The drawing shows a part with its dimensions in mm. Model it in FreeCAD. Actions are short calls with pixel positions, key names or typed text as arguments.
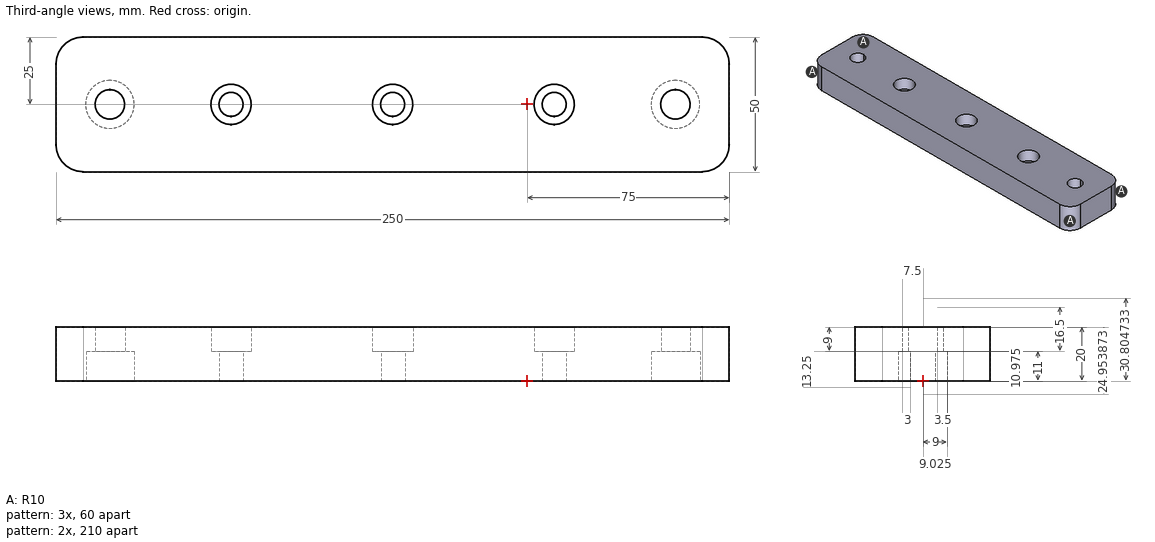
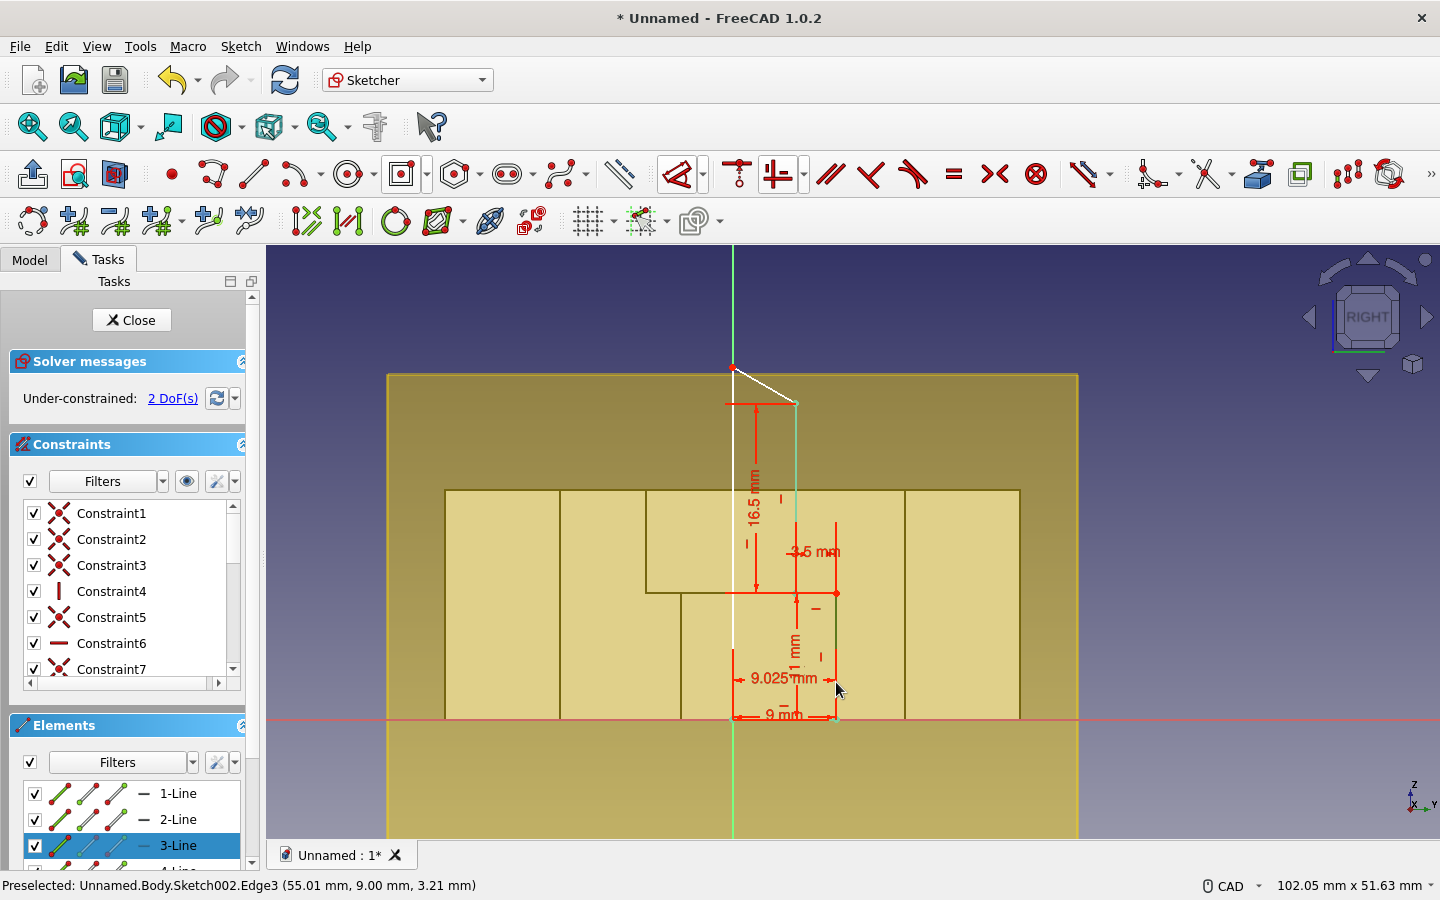
key(i)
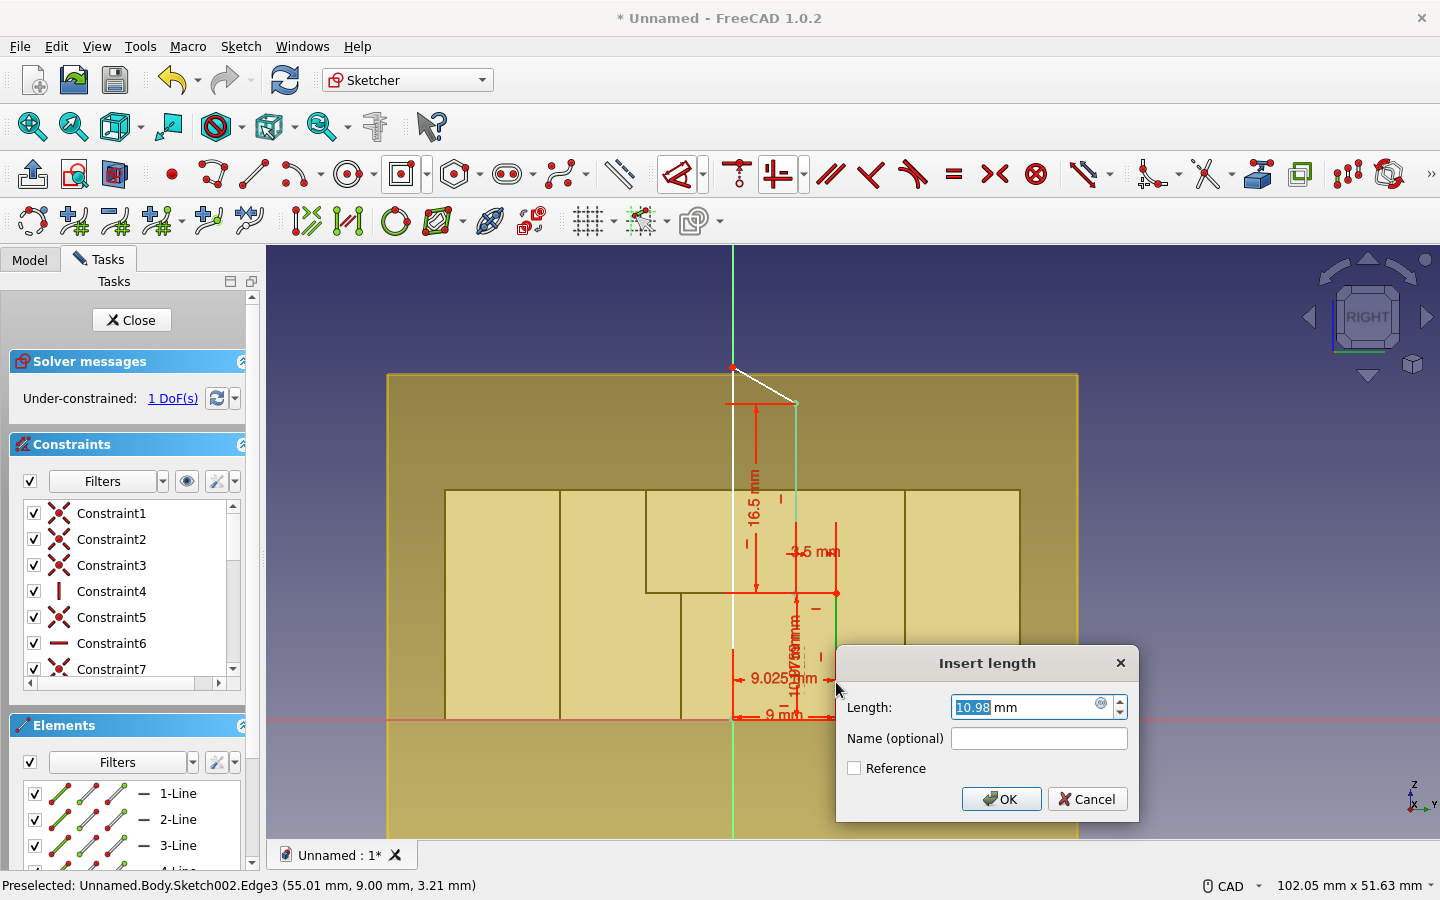
text(10.975)
key(Return)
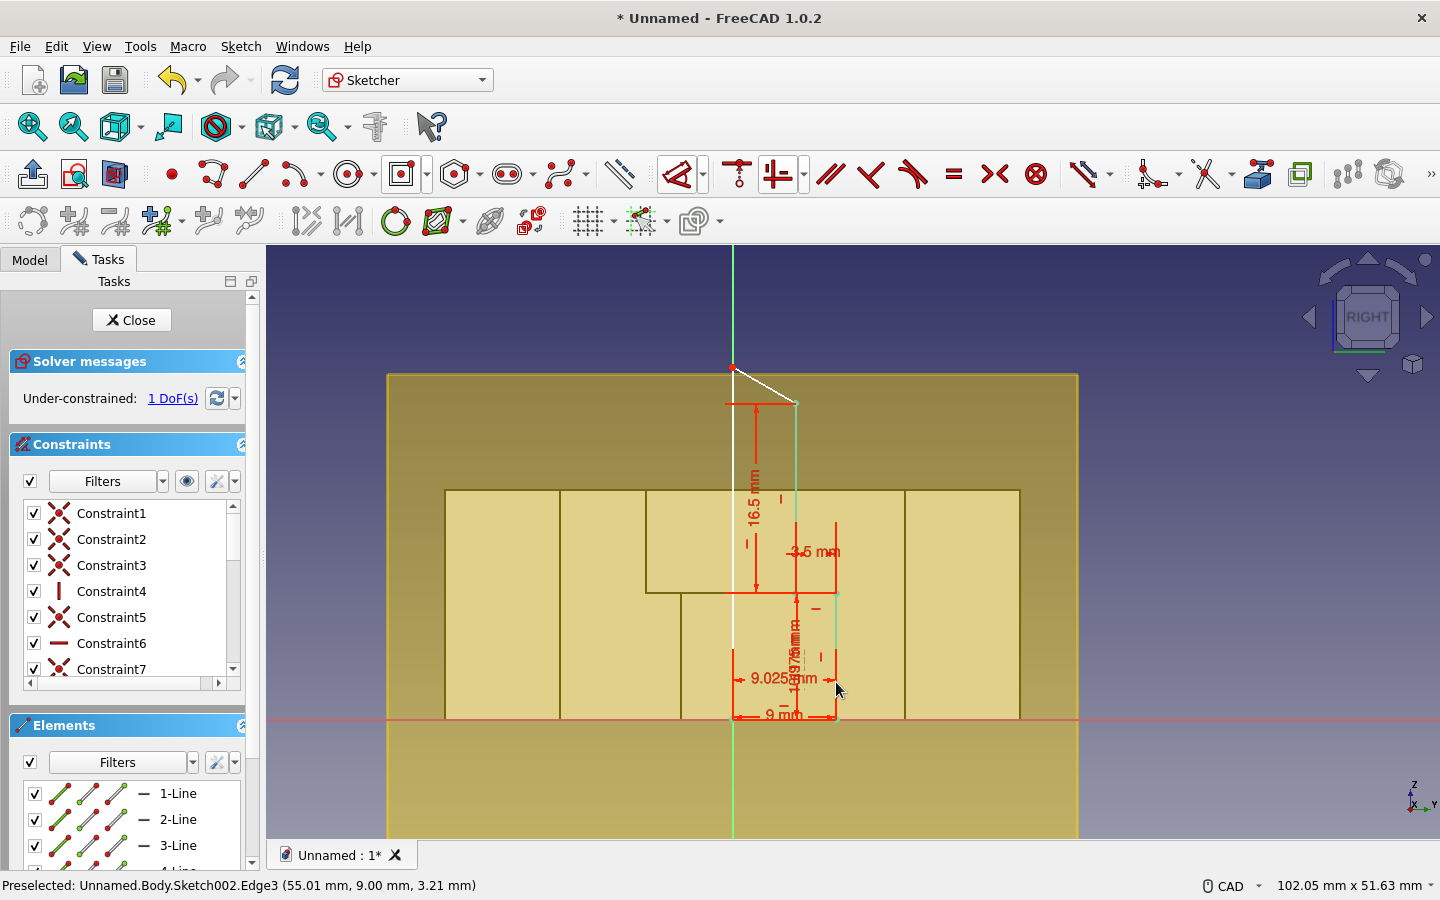
click(733, 473)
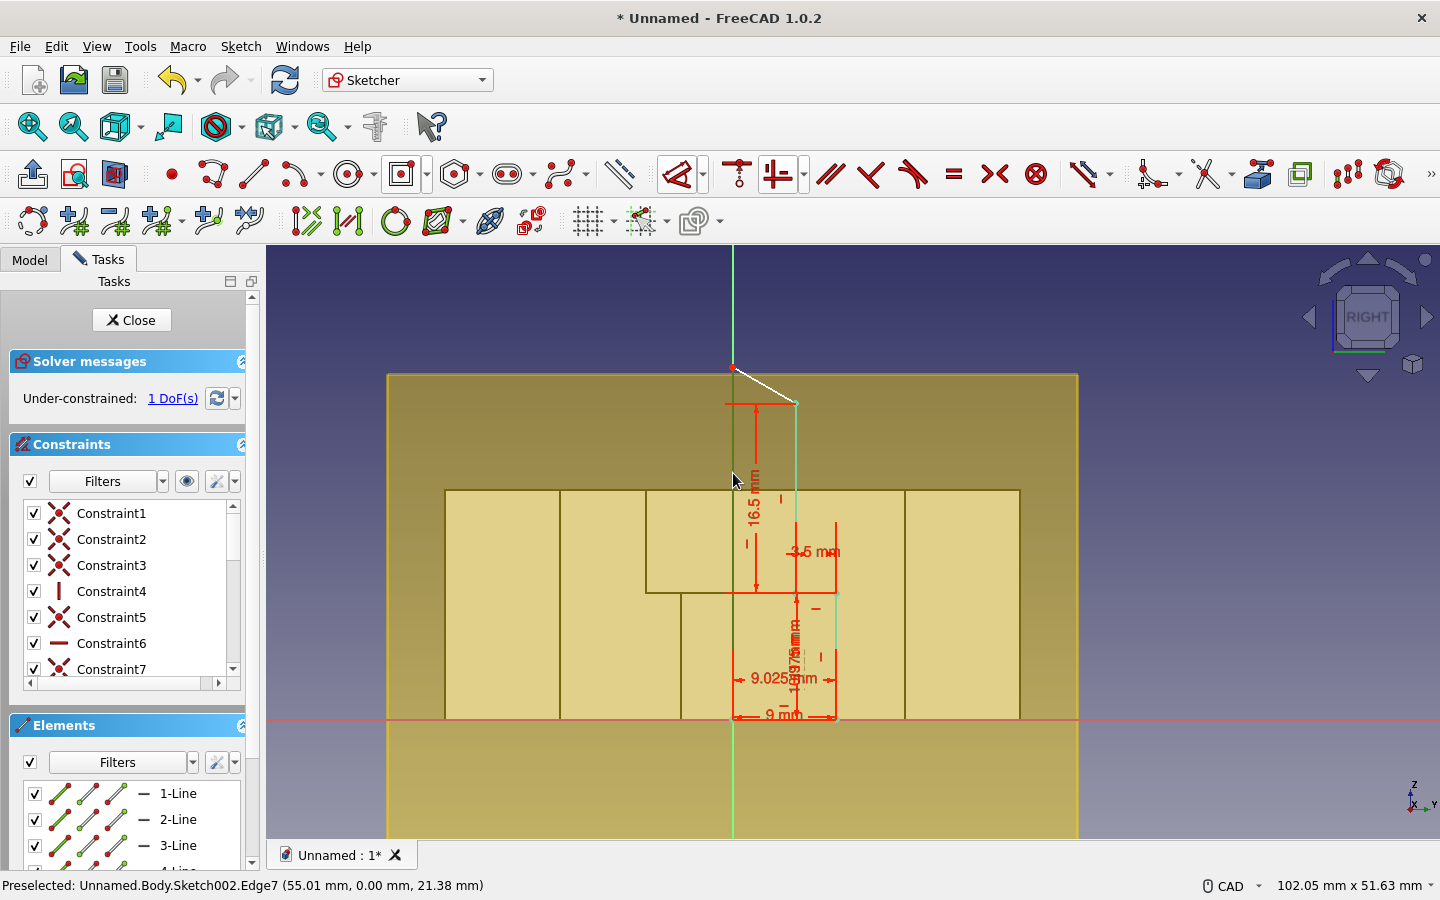
key(i)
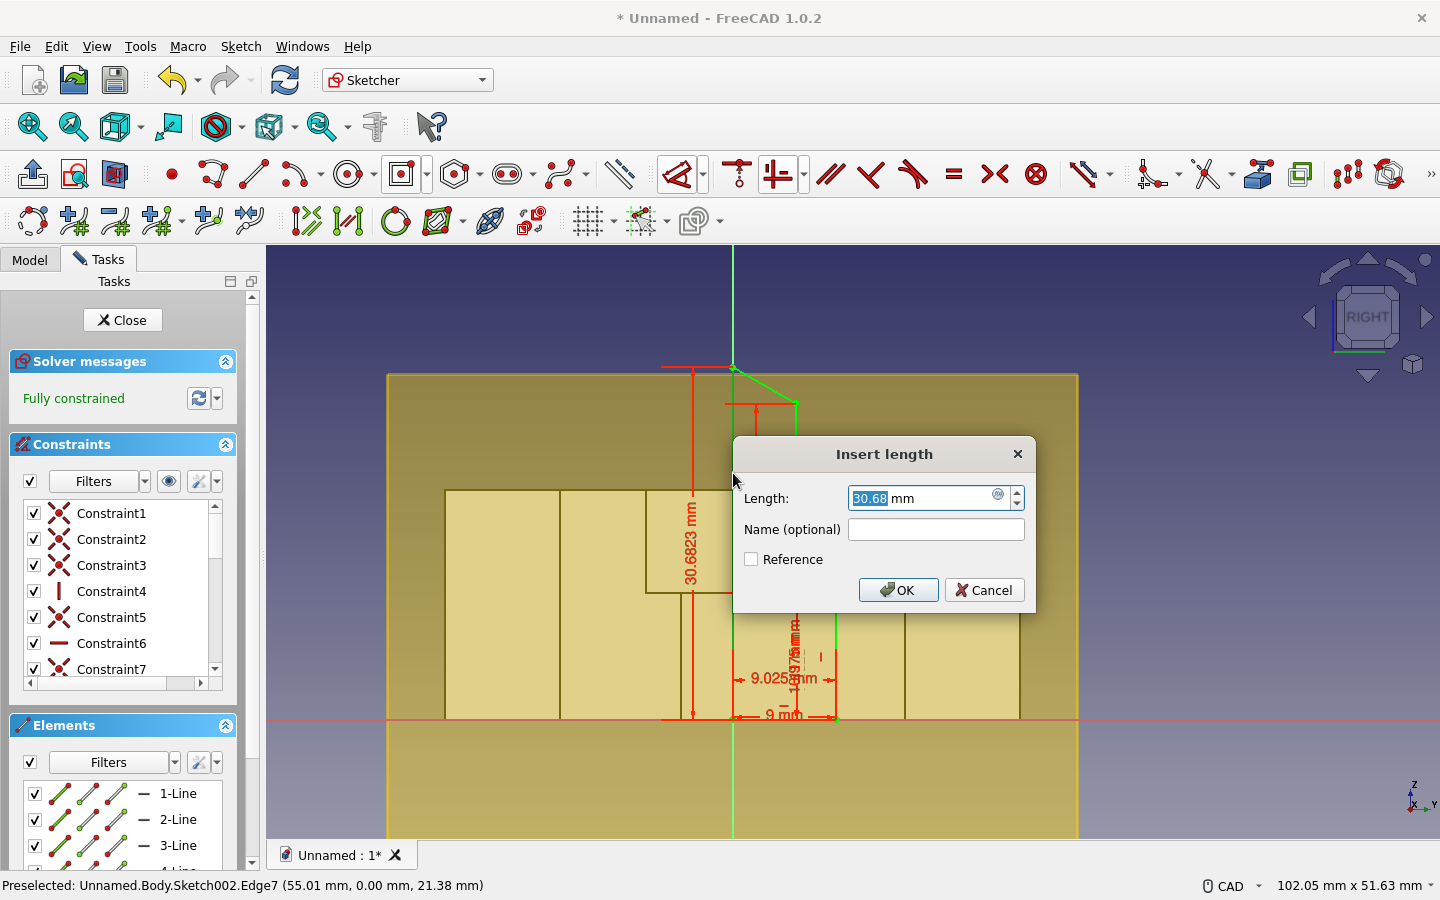
text(30.804733)
key(Return)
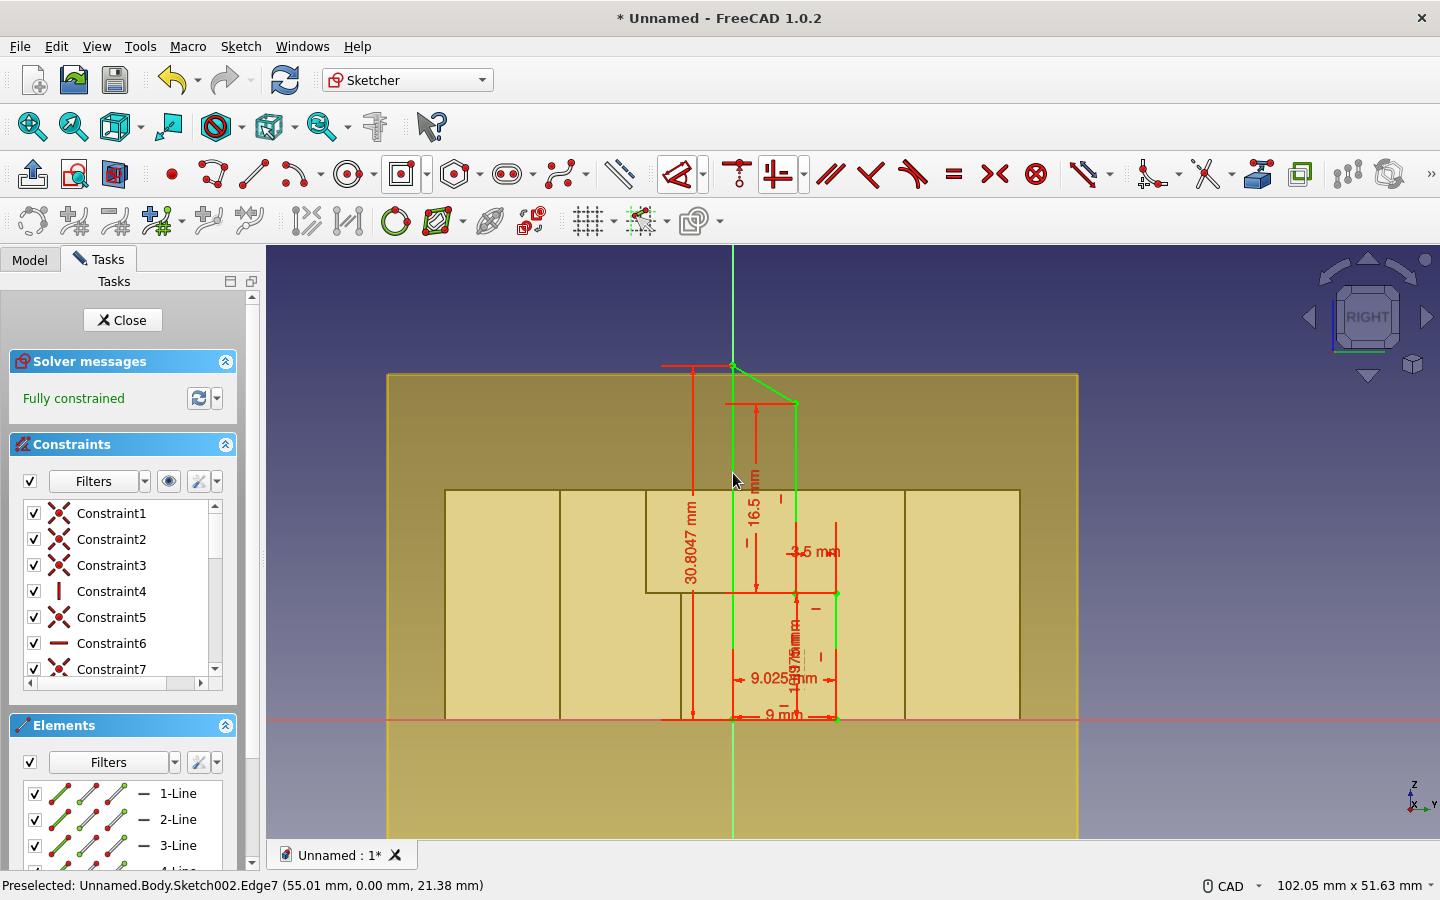
click(123, 320)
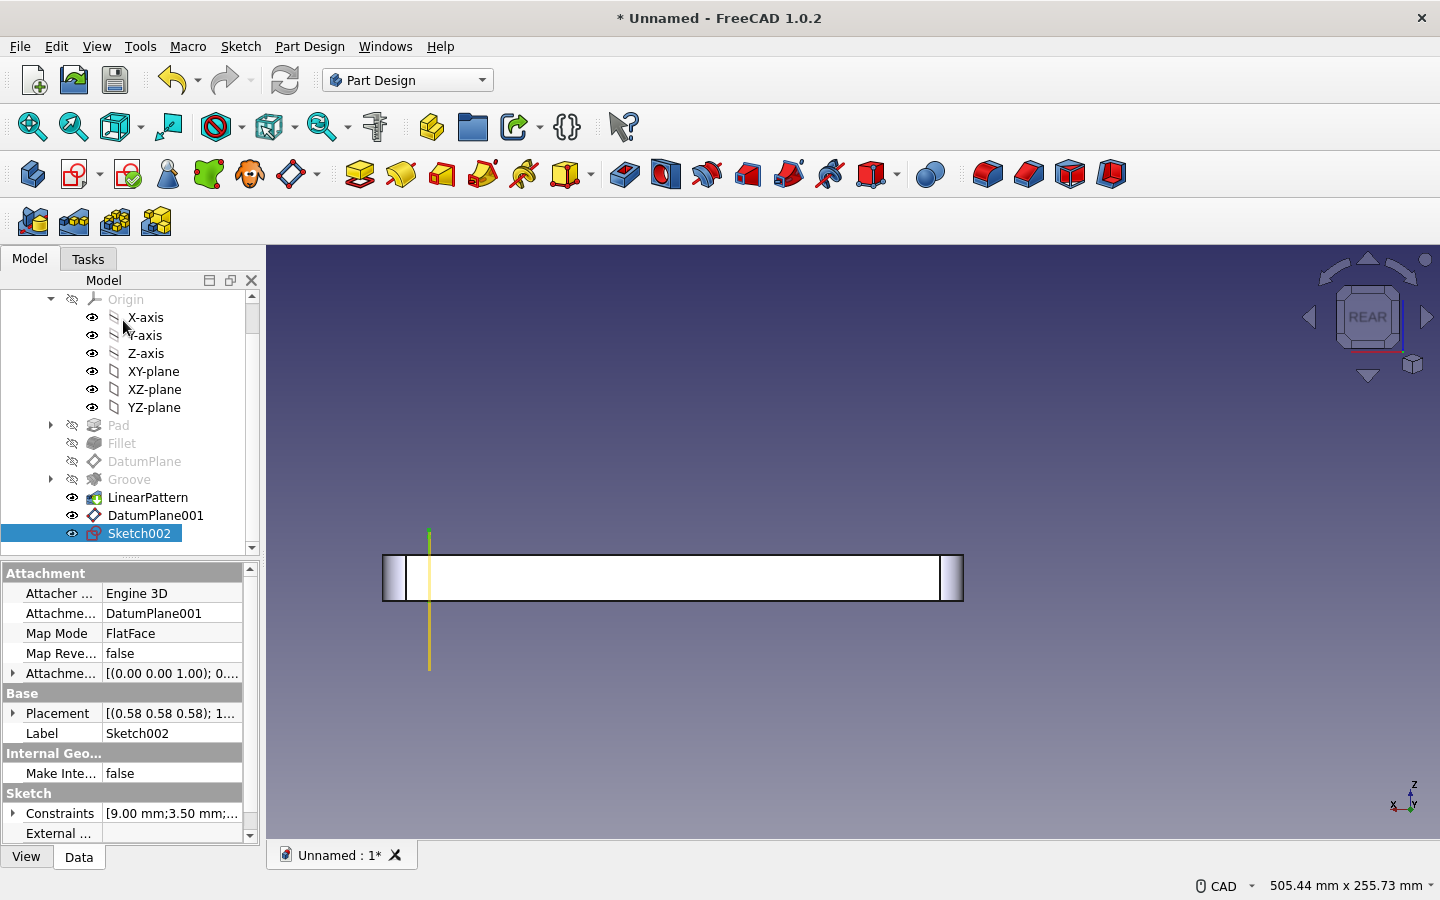
click(707, 174)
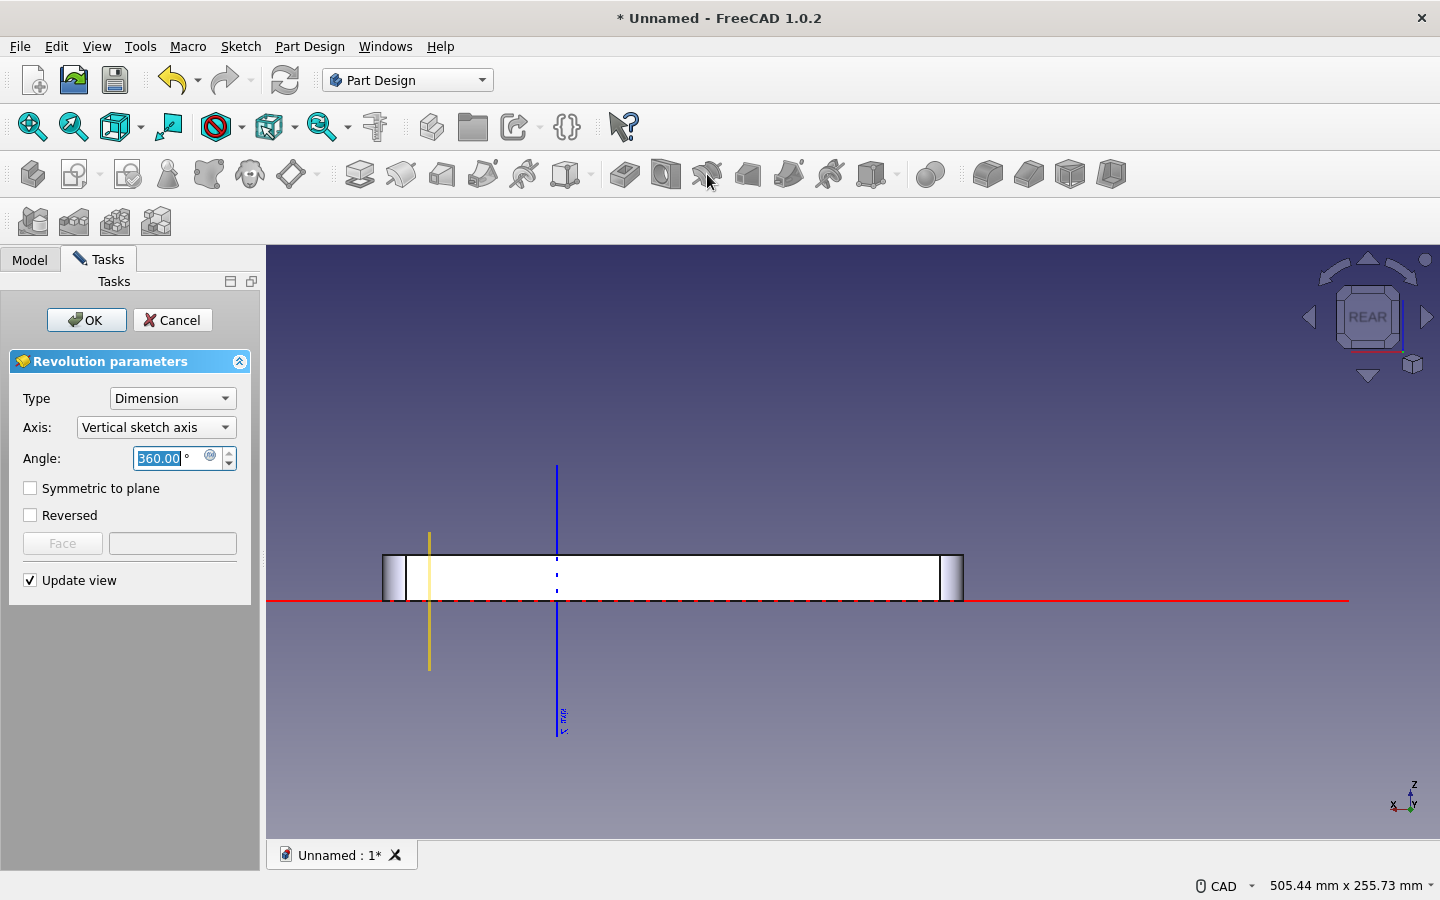
click(87, 320)